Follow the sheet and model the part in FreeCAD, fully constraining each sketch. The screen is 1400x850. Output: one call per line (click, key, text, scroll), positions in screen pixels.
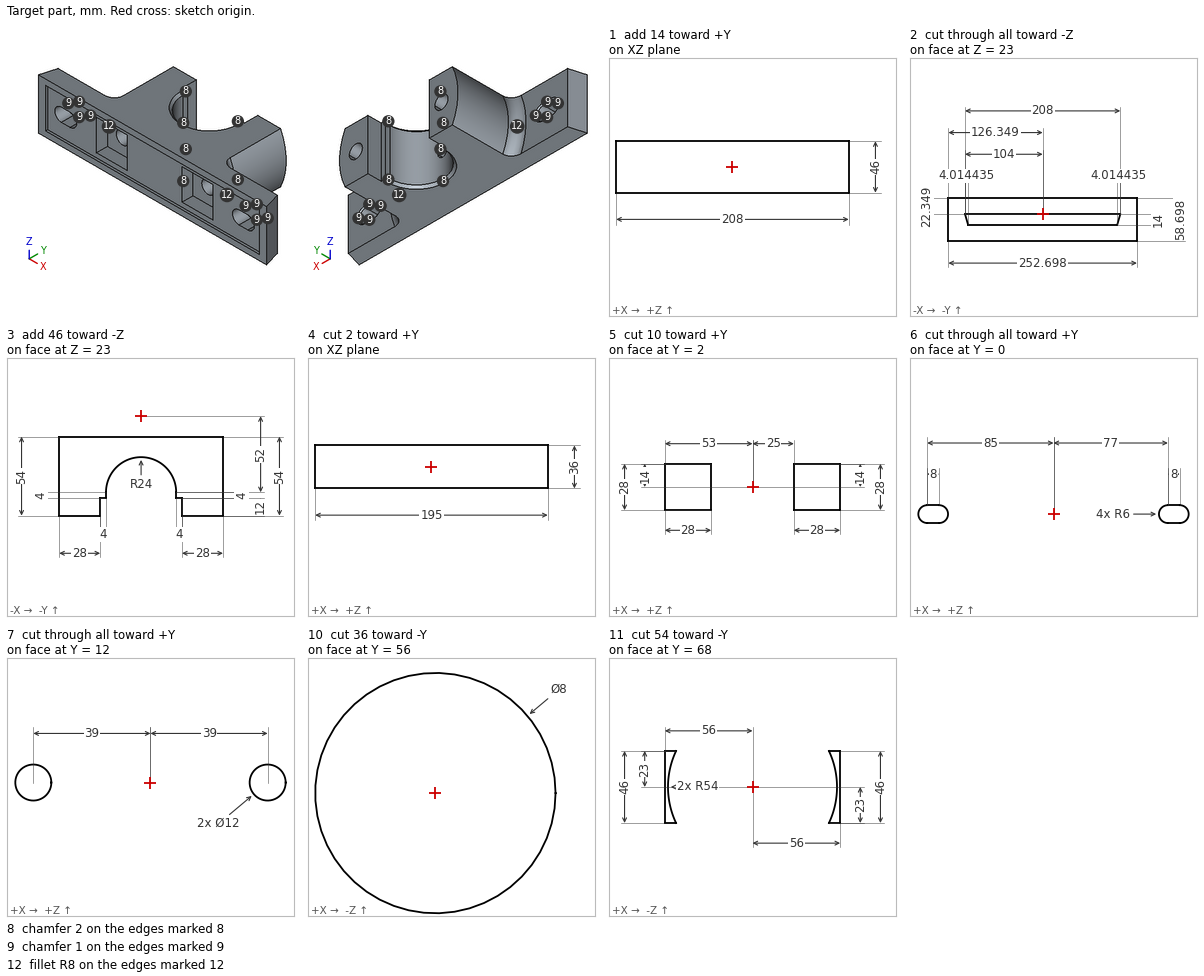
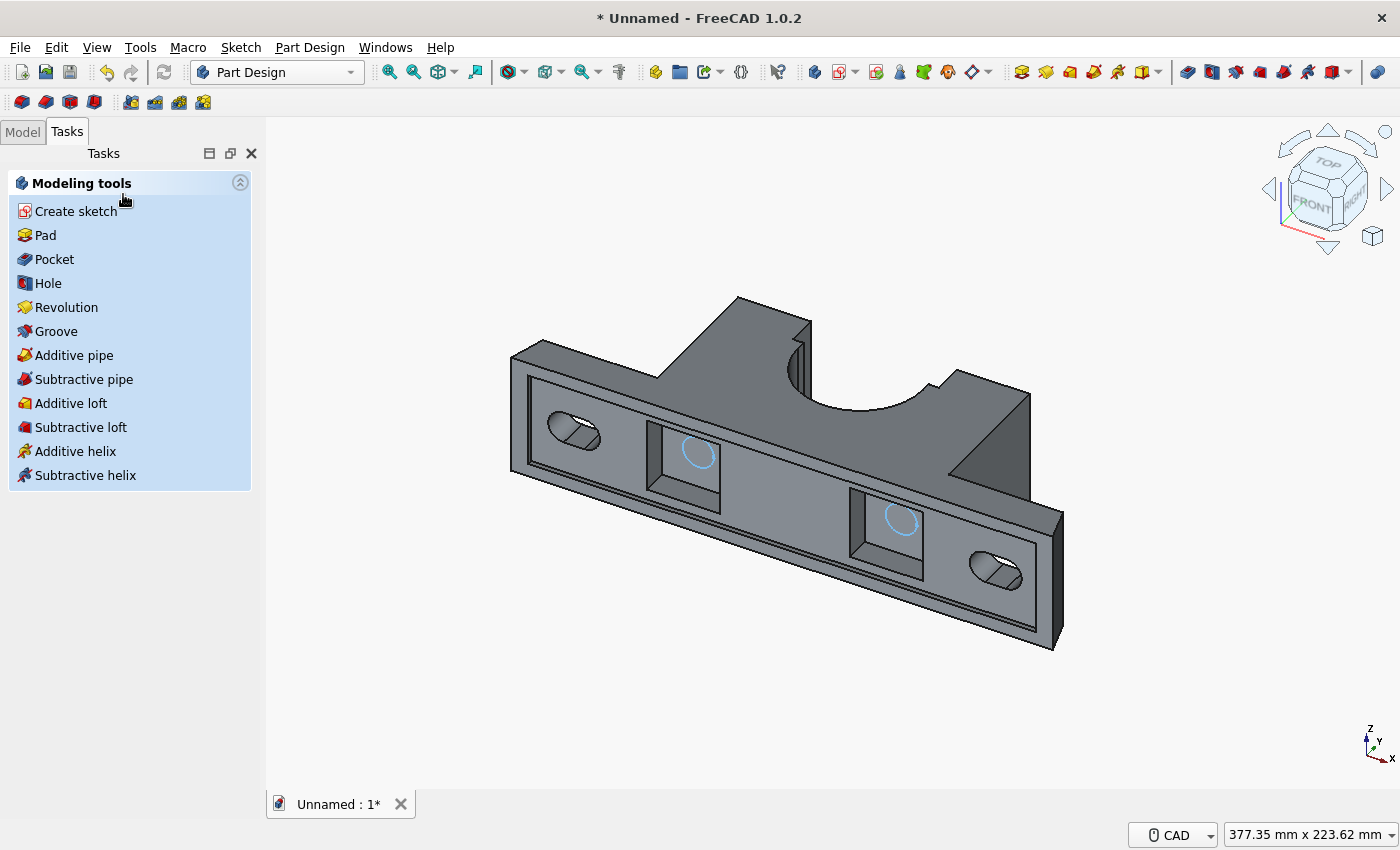
click(1188, 72)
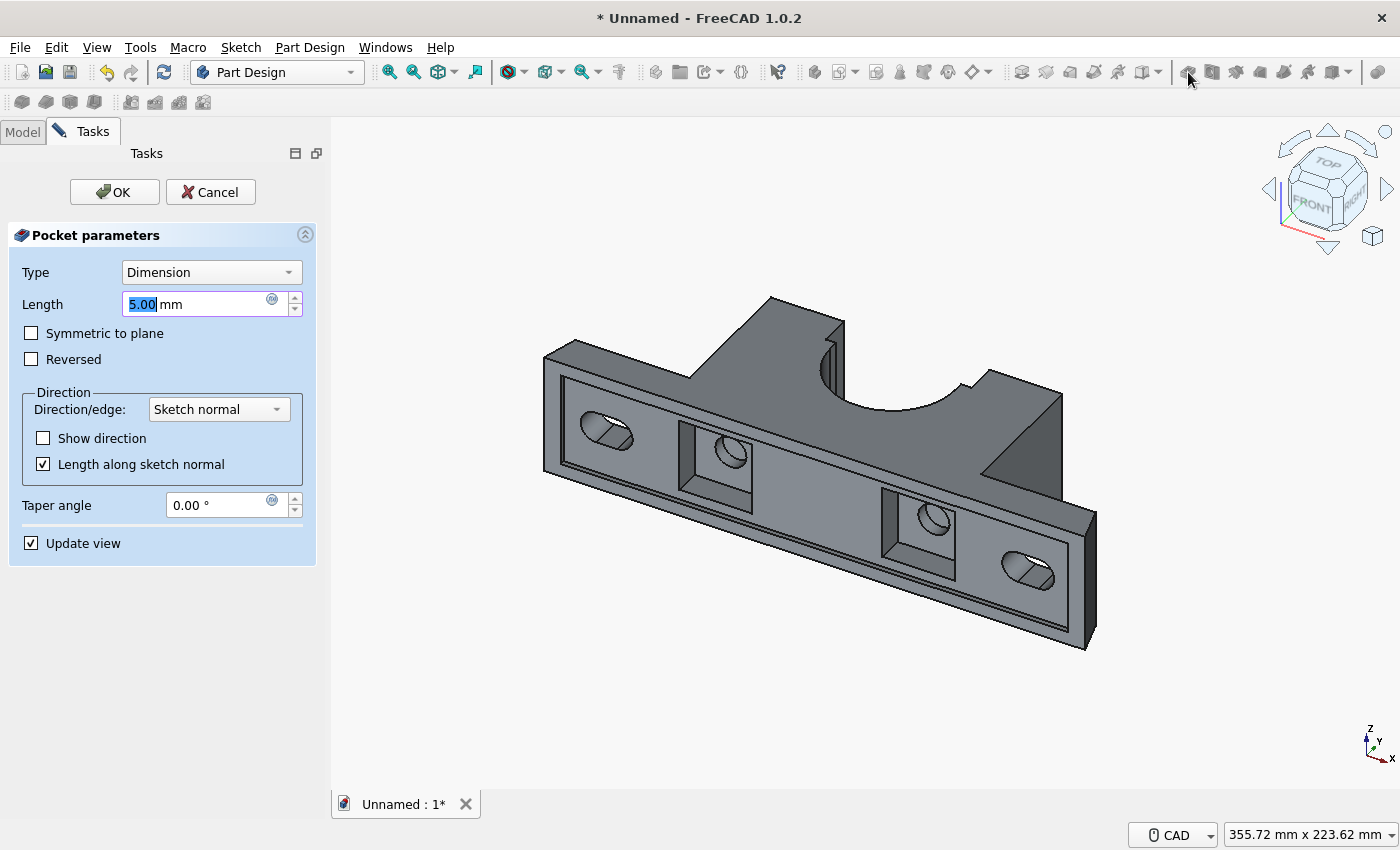
click(212, 272)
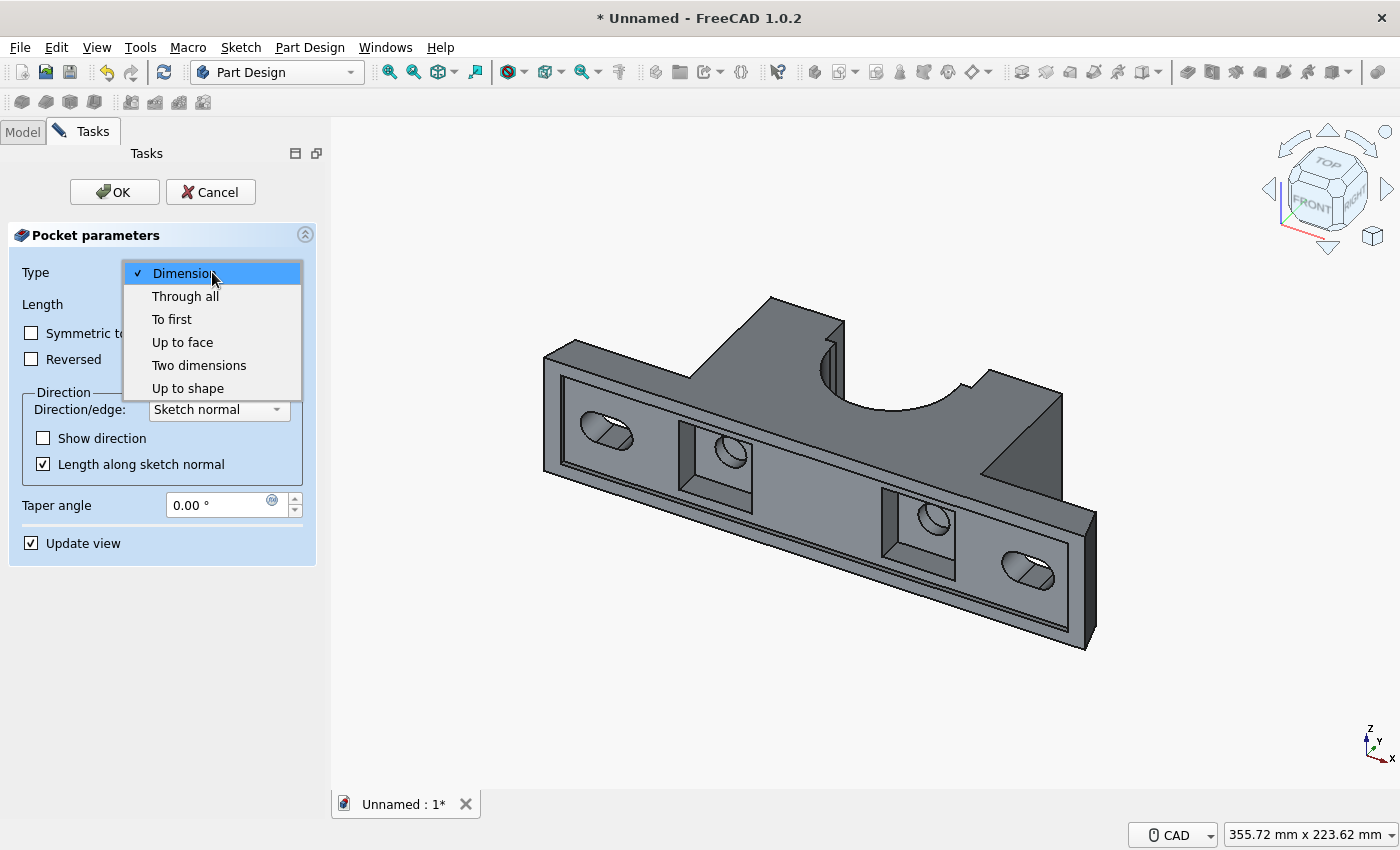
click(212, 296)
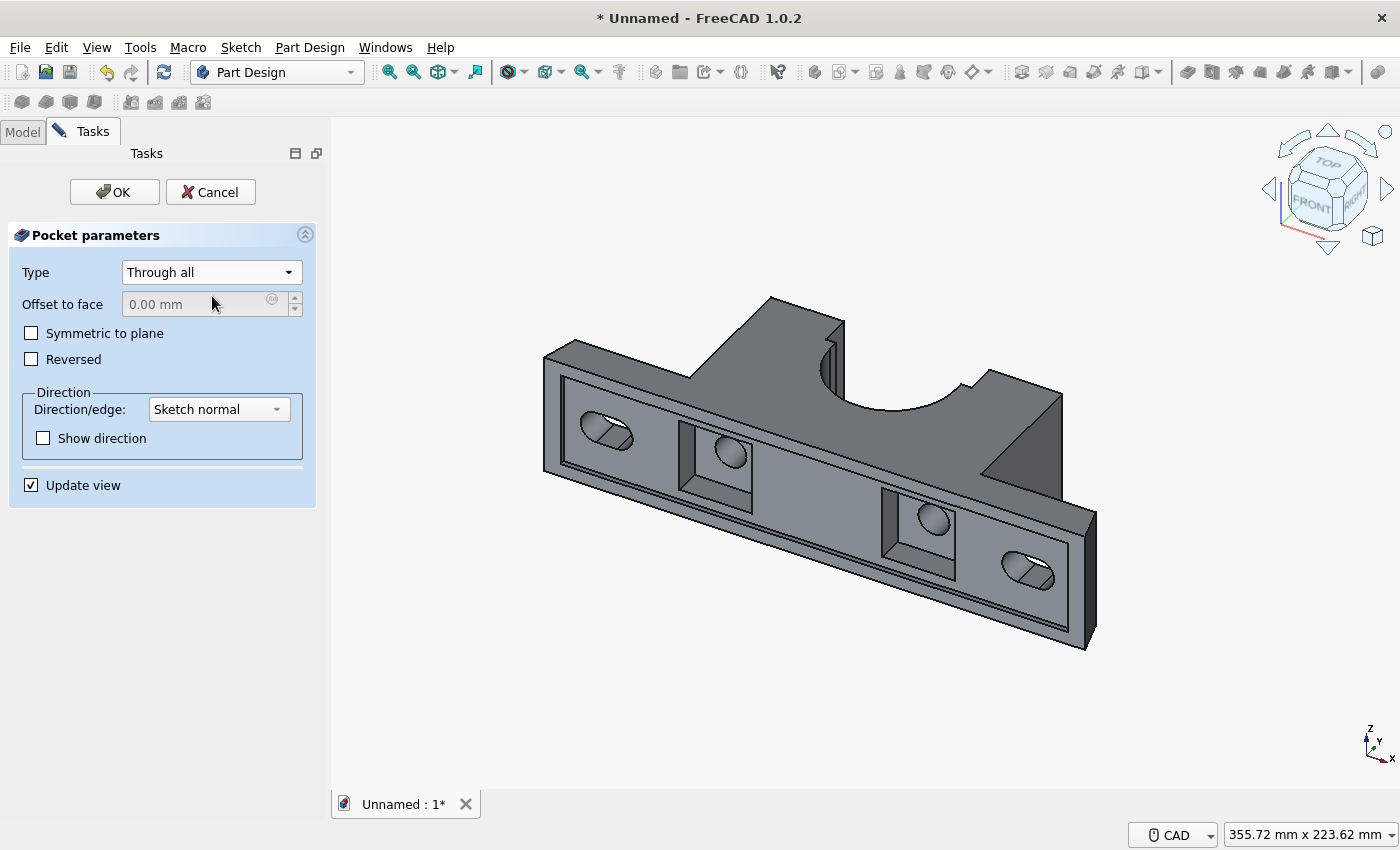
click(115, 192)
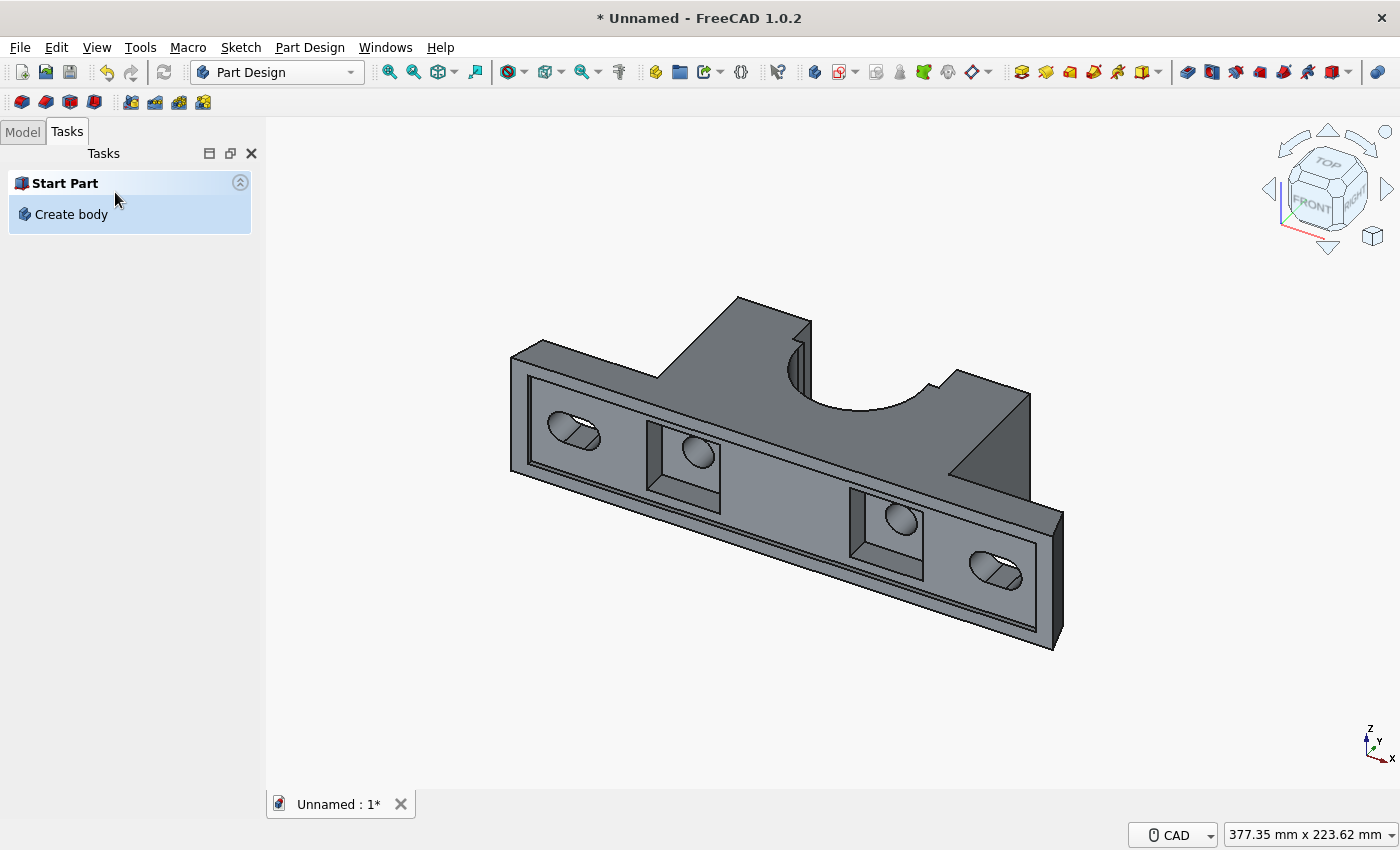
click(806, 396)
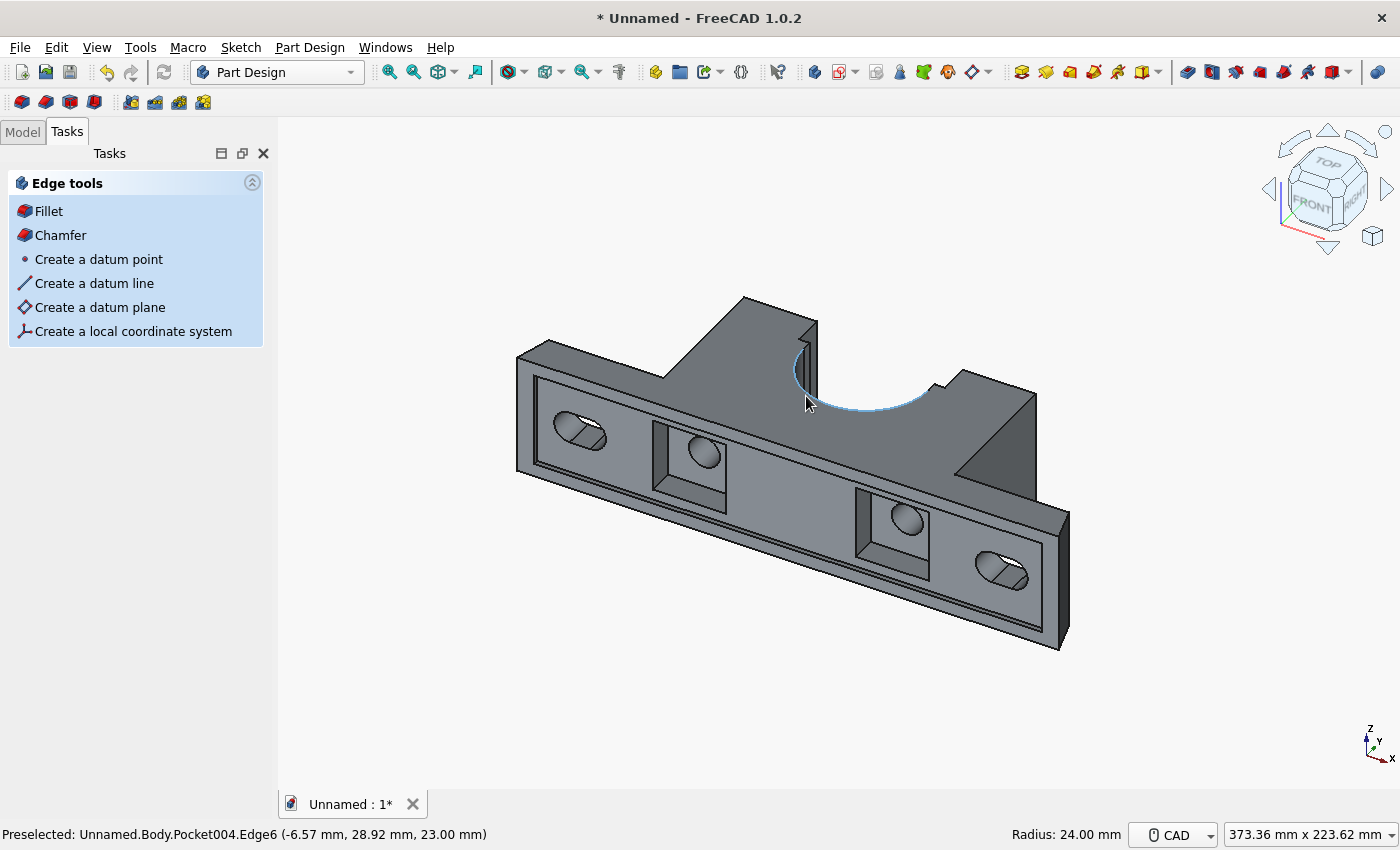
click(808, 343, ctrl)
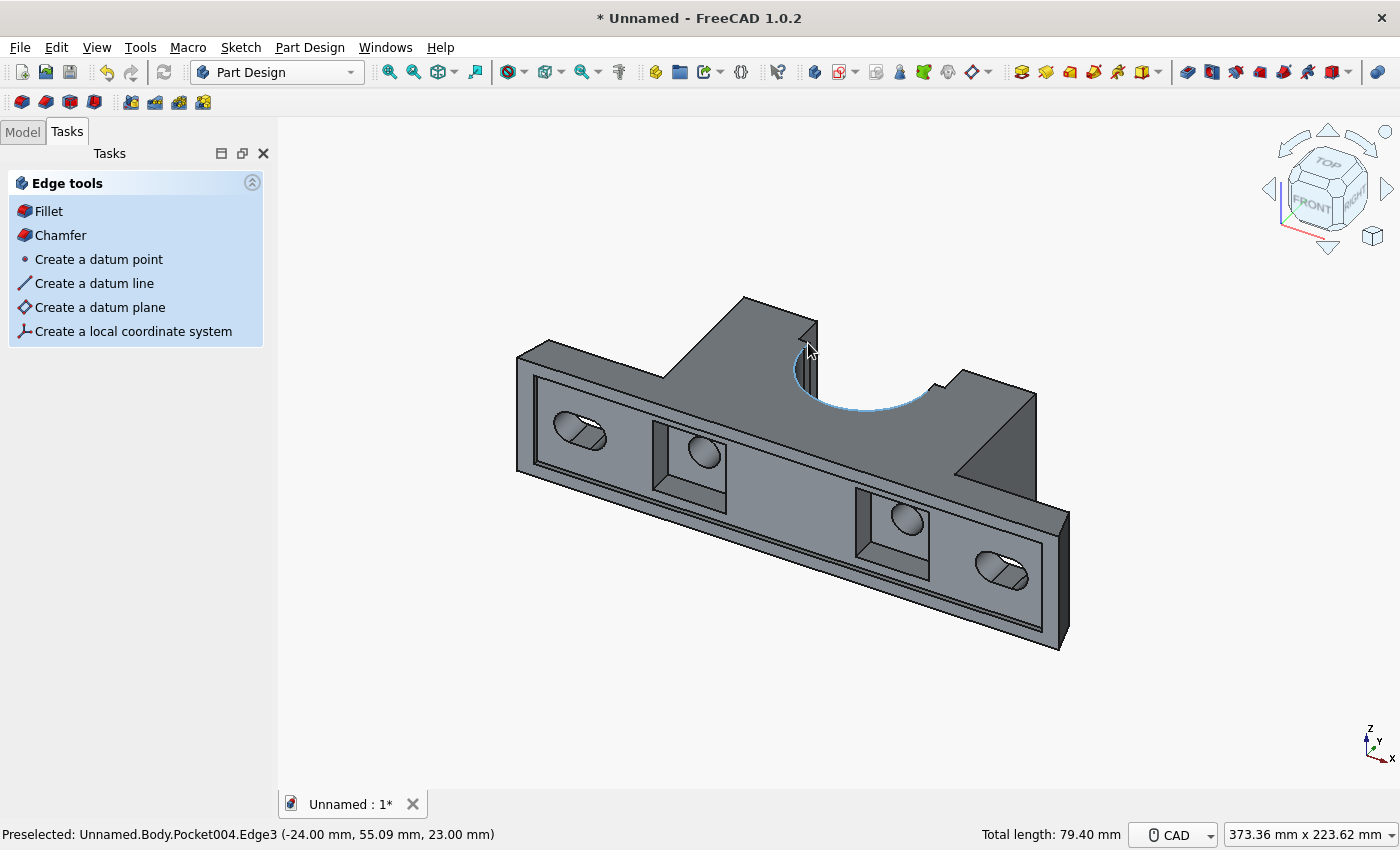
scroll(807, 458, up, 7)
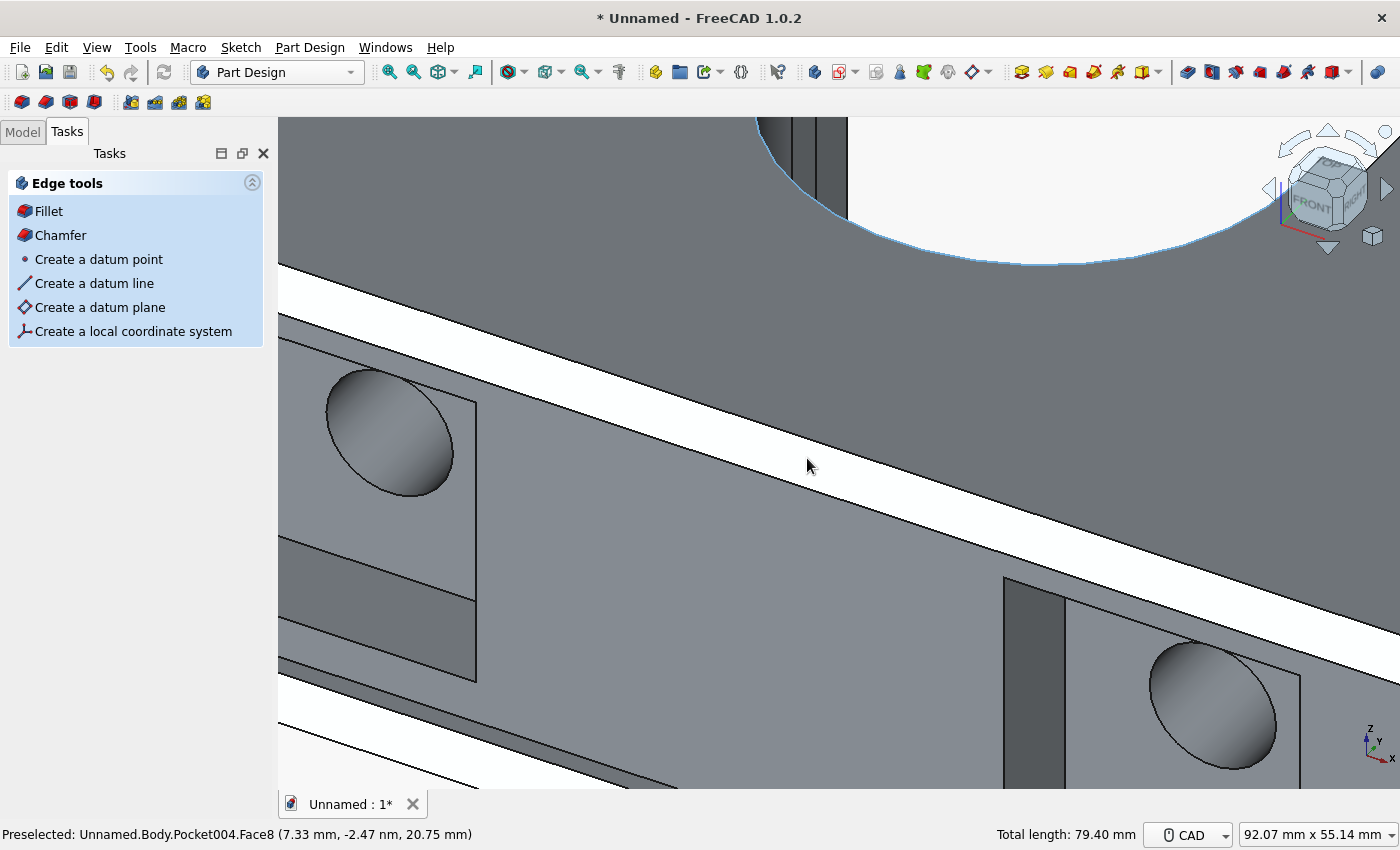
key(v)
key(f)